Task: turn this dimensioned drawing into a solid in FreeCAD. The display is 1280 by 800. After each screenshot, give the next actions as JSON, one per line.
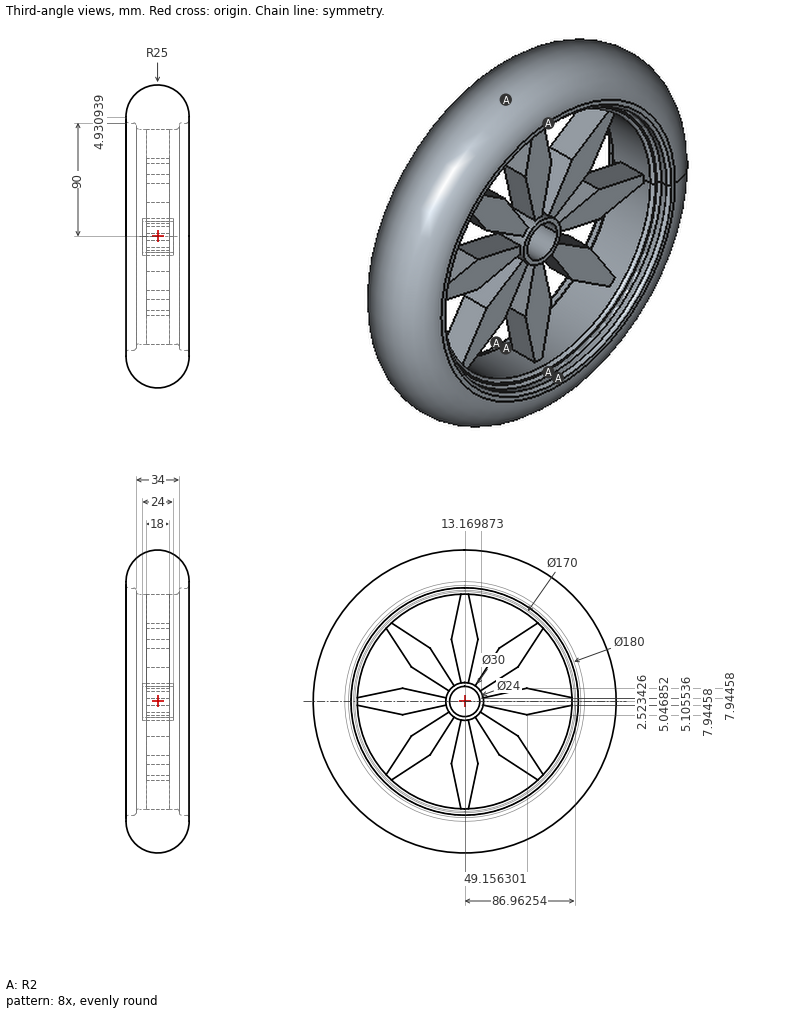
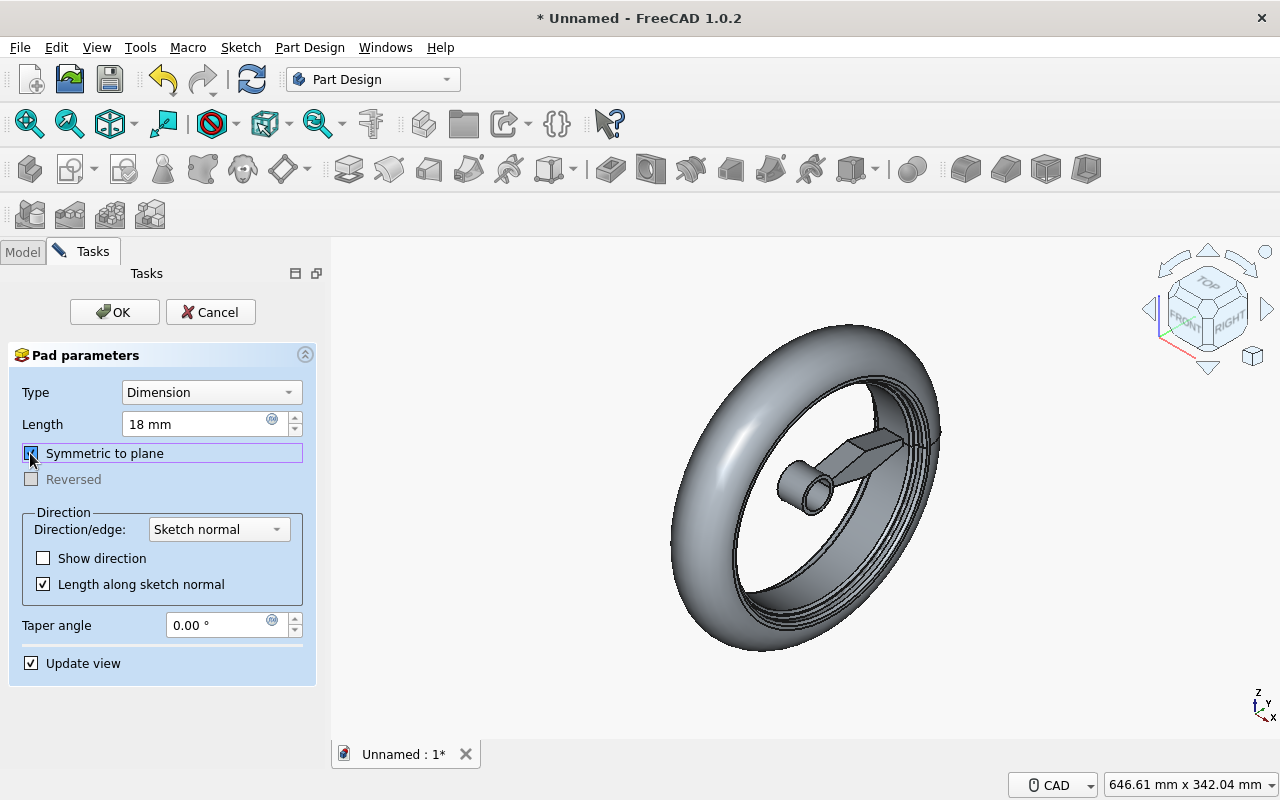
{"action": "left_click", "coordinate": [115, 312]}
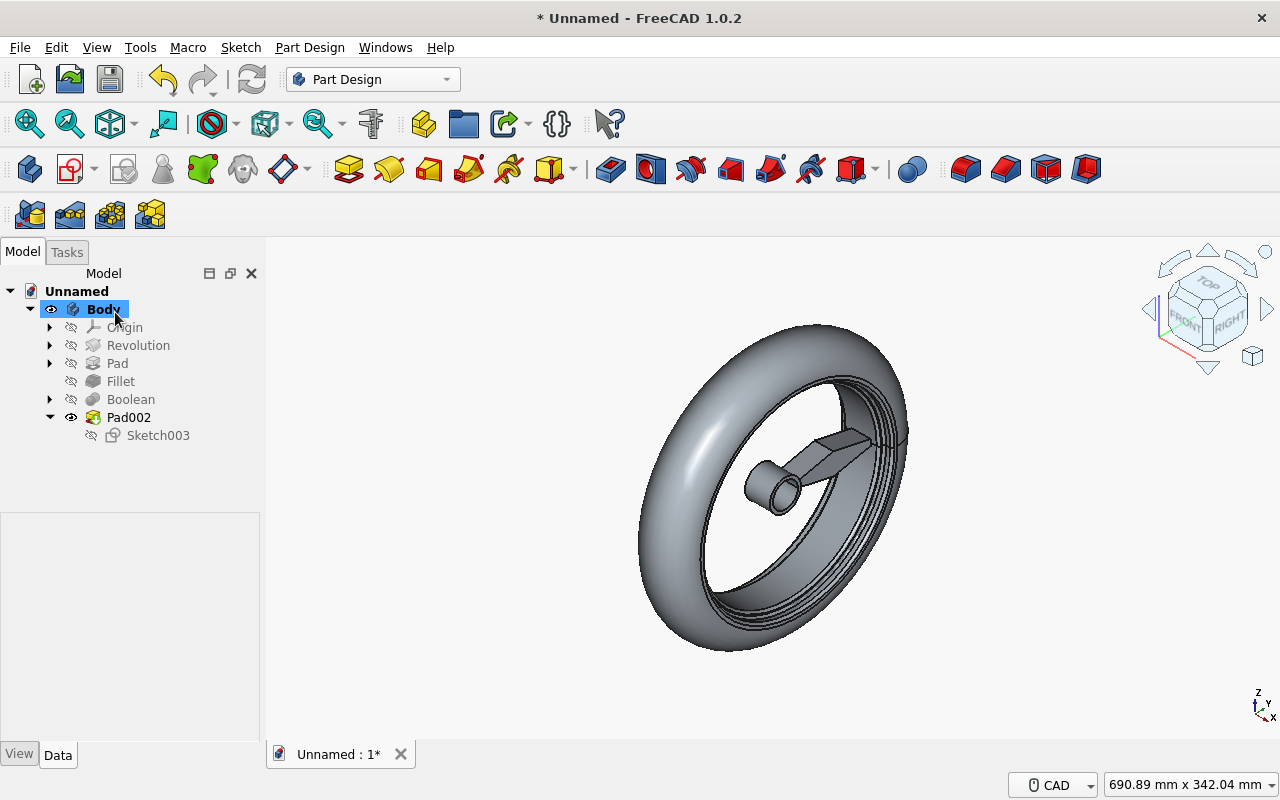
{"action": "left_click", "coordinate": [116, 417]}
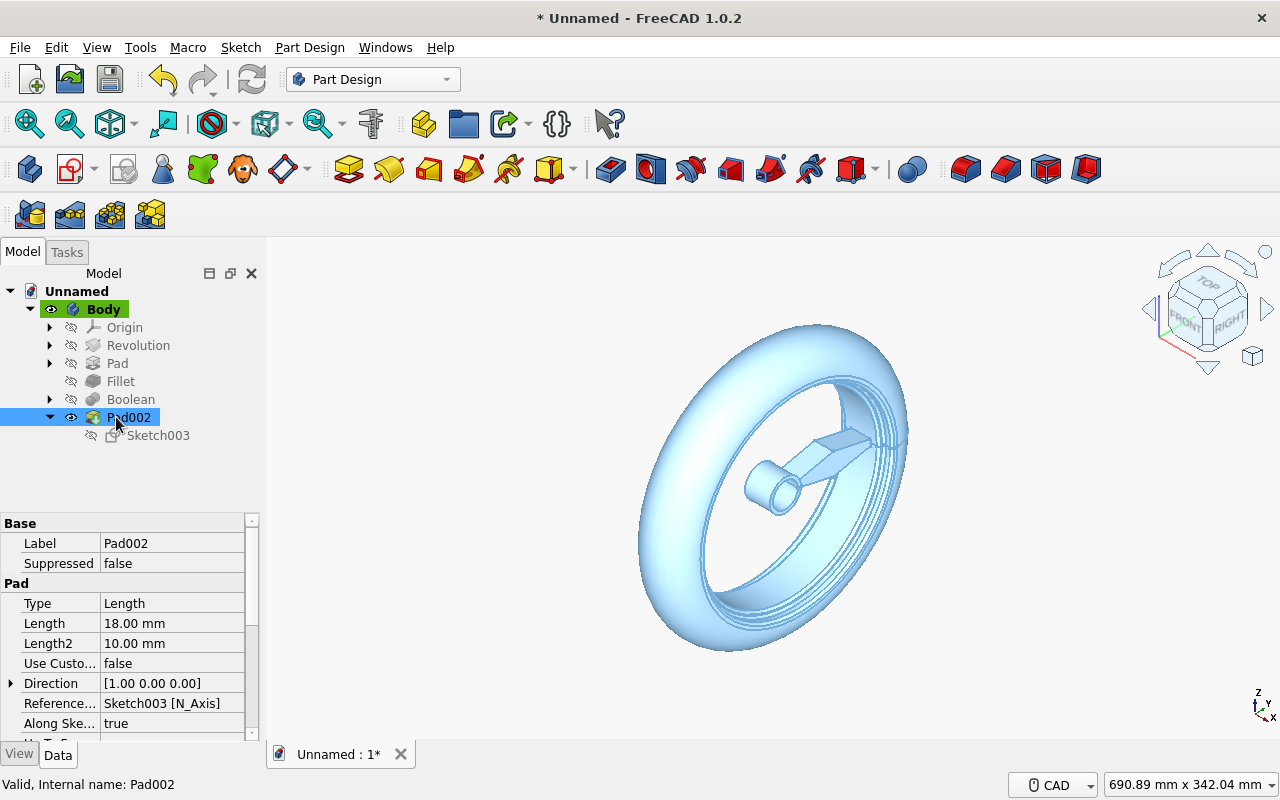
{"action": "left_click", "coordinate": [110, 214]}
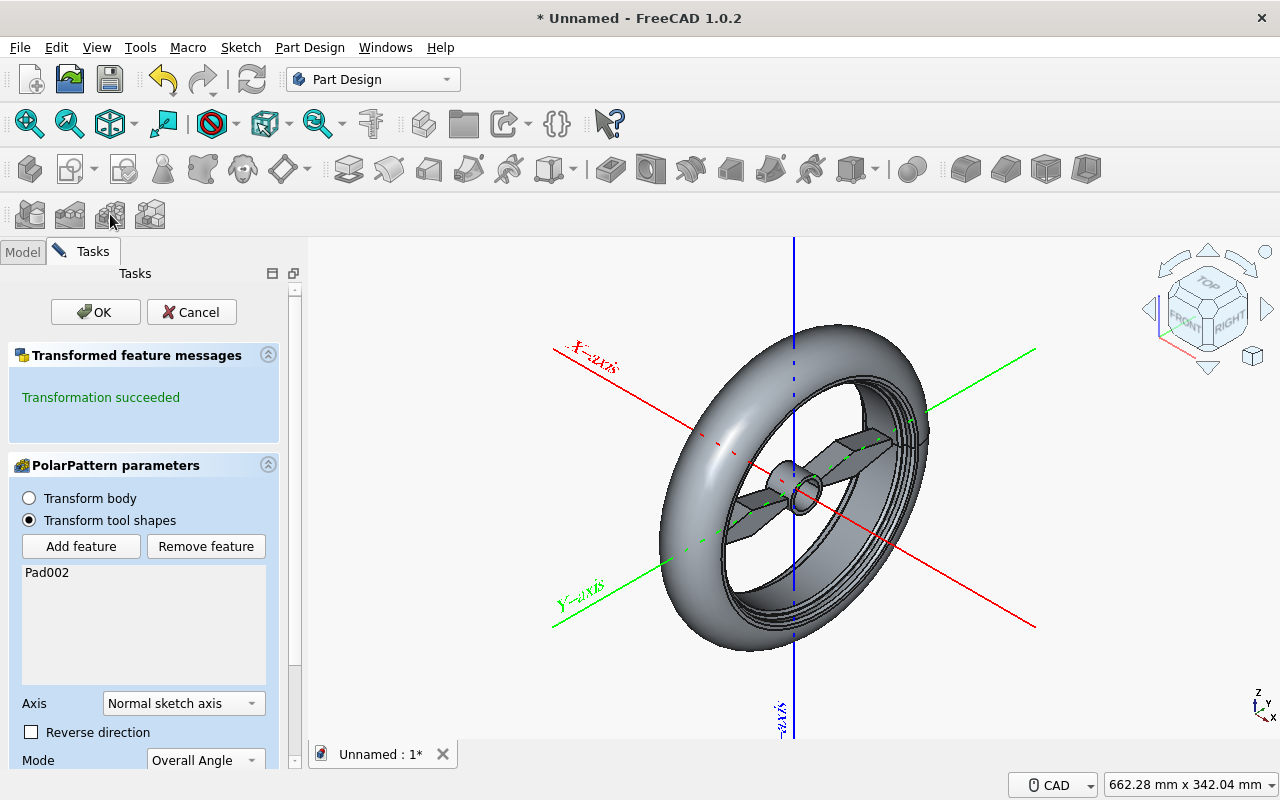
{"action": "left_click", "coordinate": [184, 704]}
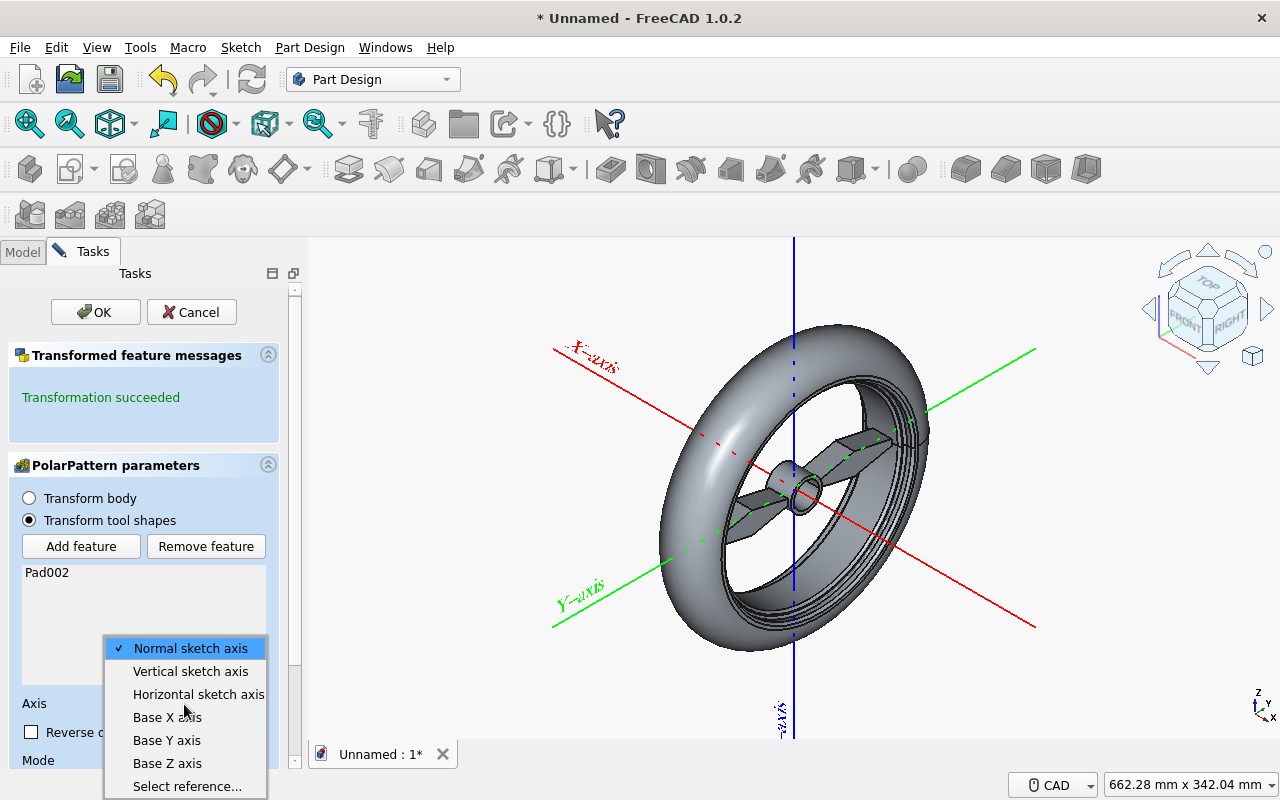
{"action": "left_click", "coordinate": [184, 718]}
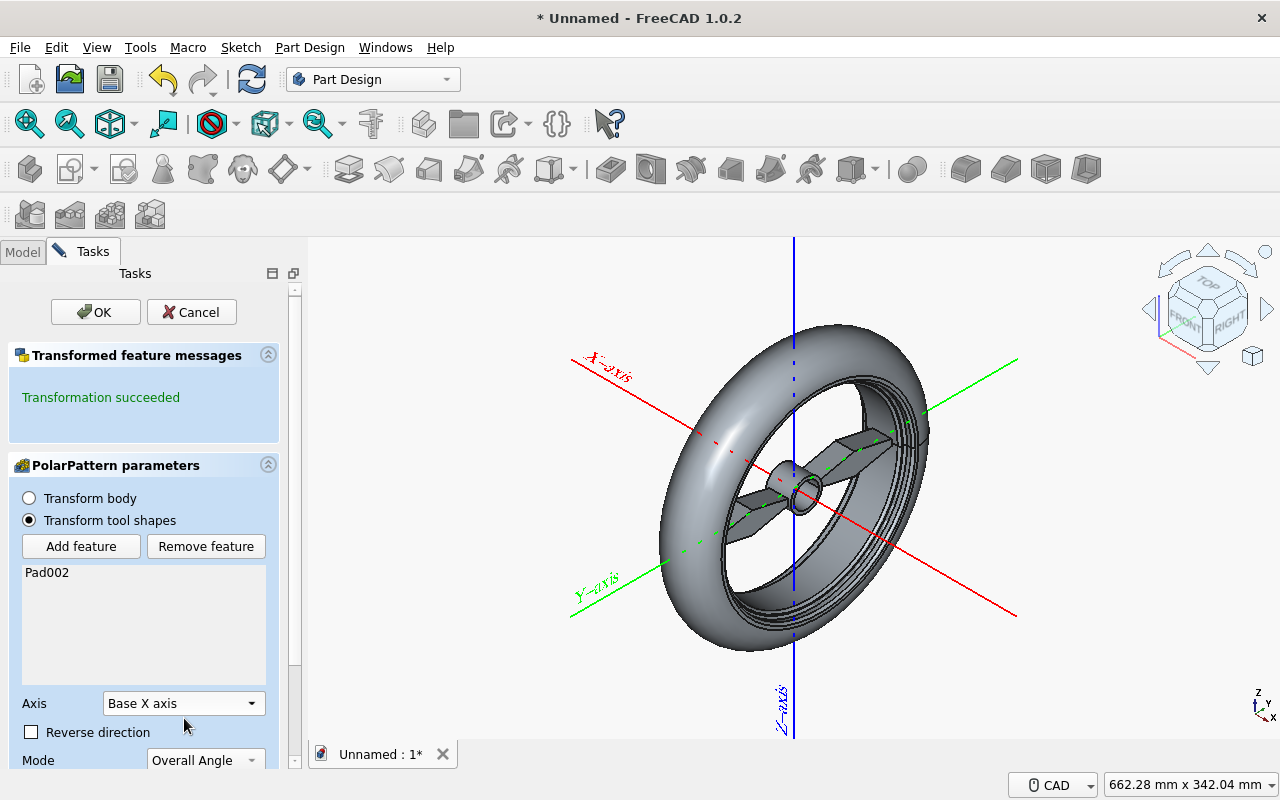
{"action": "scroll", "coordinate": [295, 526], "scroll_direction": "down", "scroll_amount": 3}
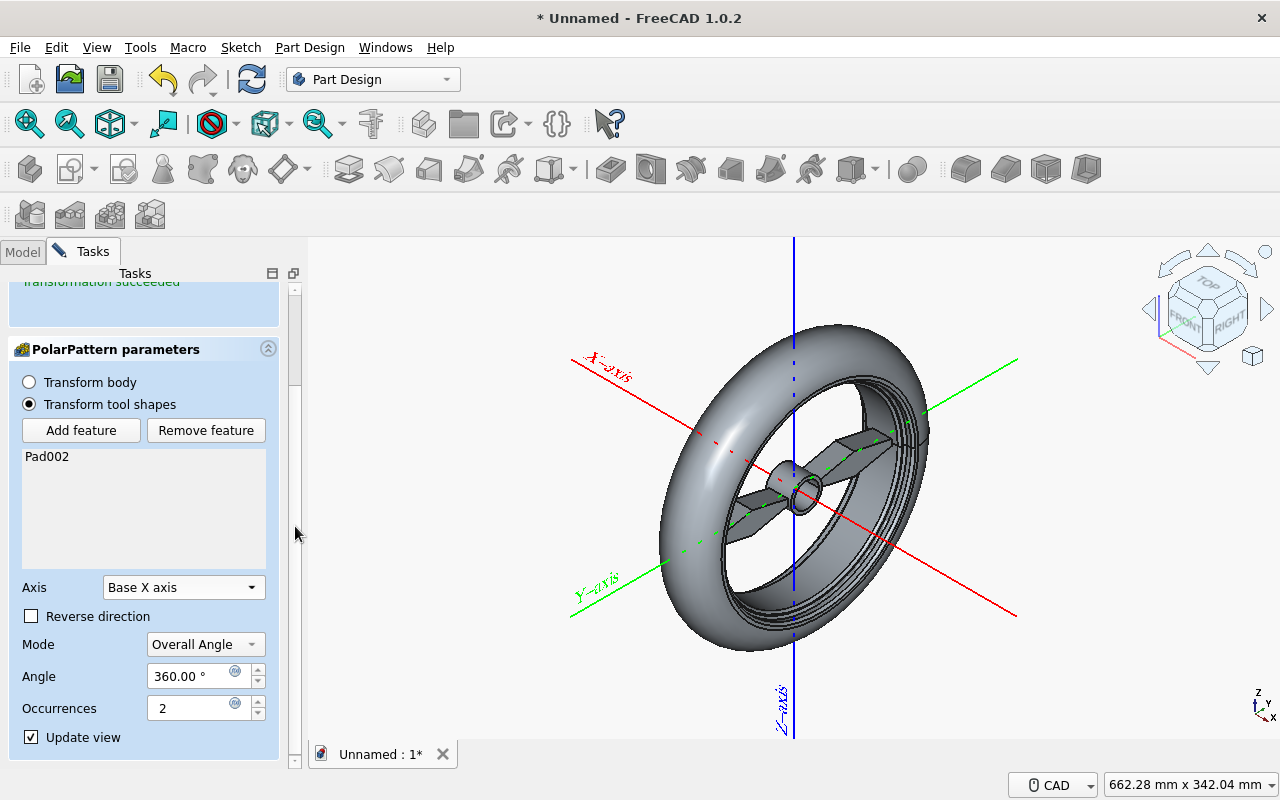
{"action": "triple_click", "coordinate": [198, 708]}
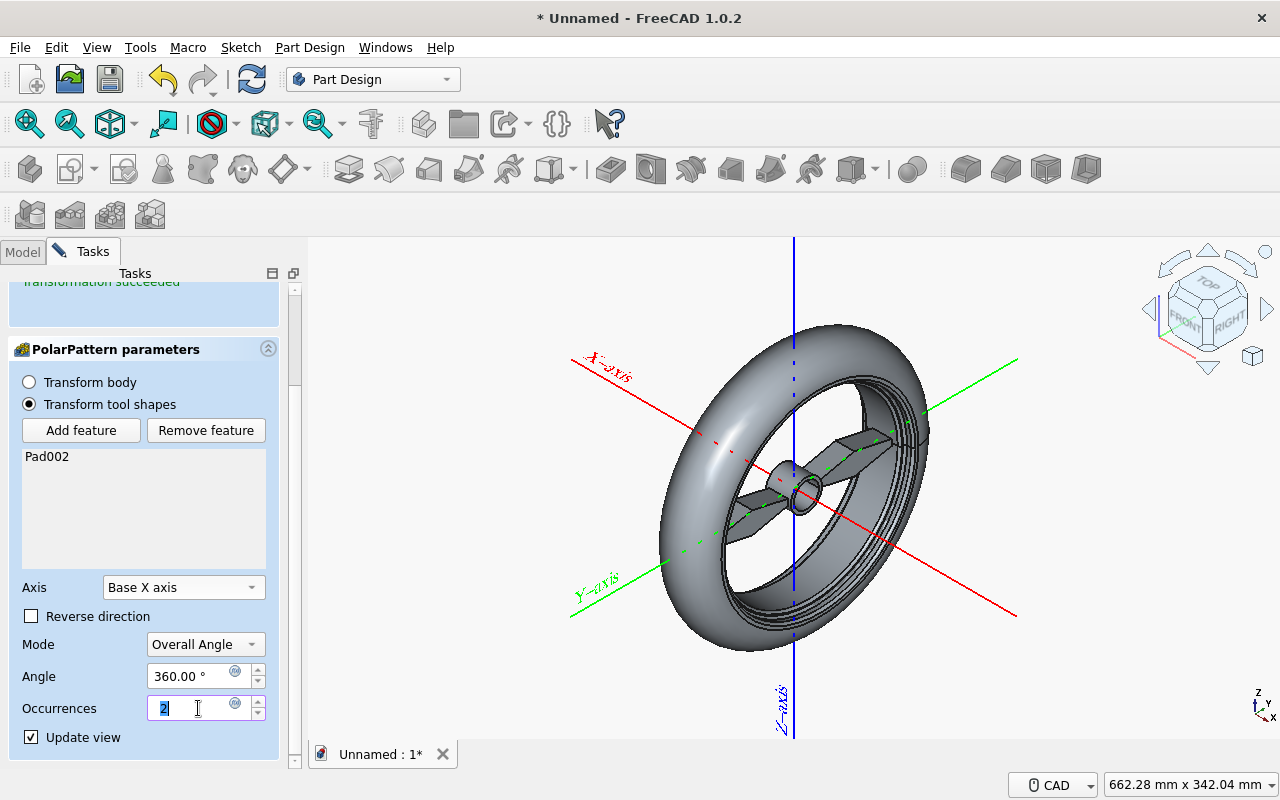
{"action": "type", "text": "8"}
{"action": "key", "text": "Tab"}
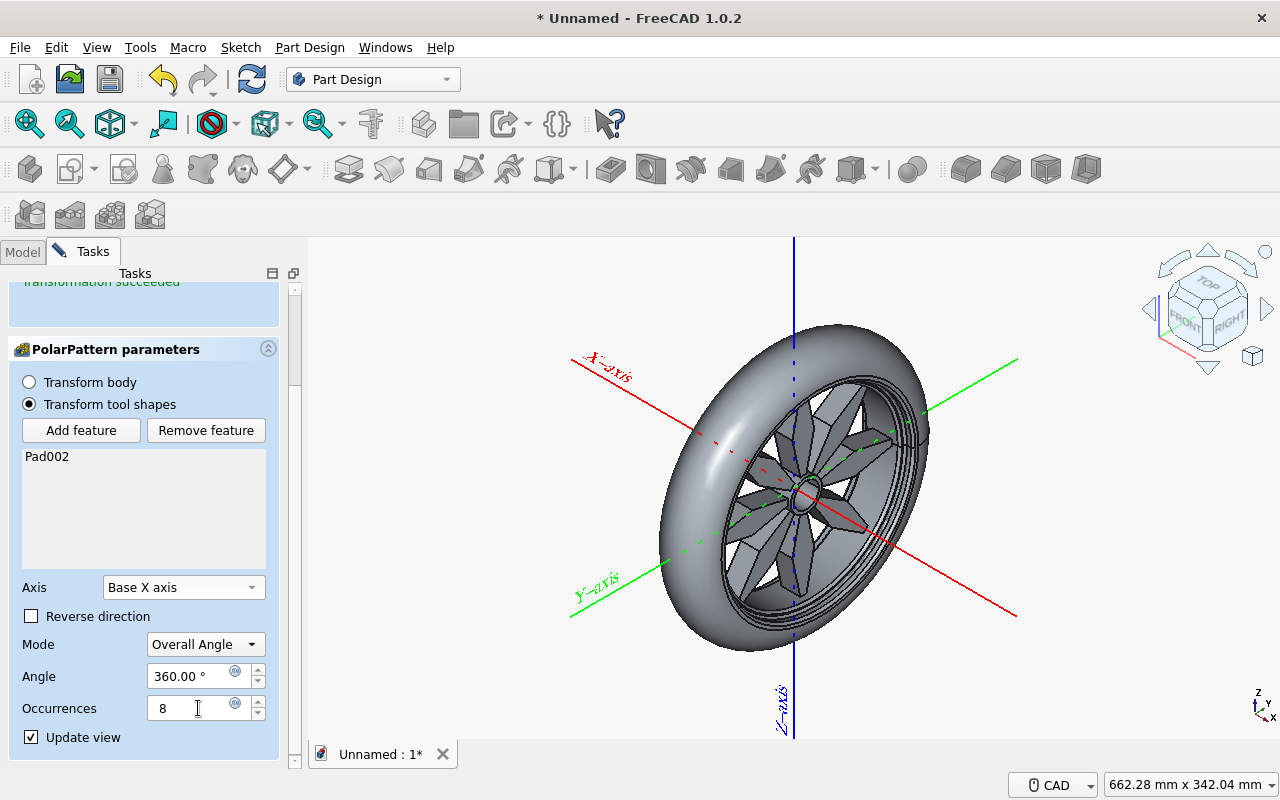
{"action": "scroll", "coordinate": [295, 526], "scroll_direction": "up", "scroll_amount": 3}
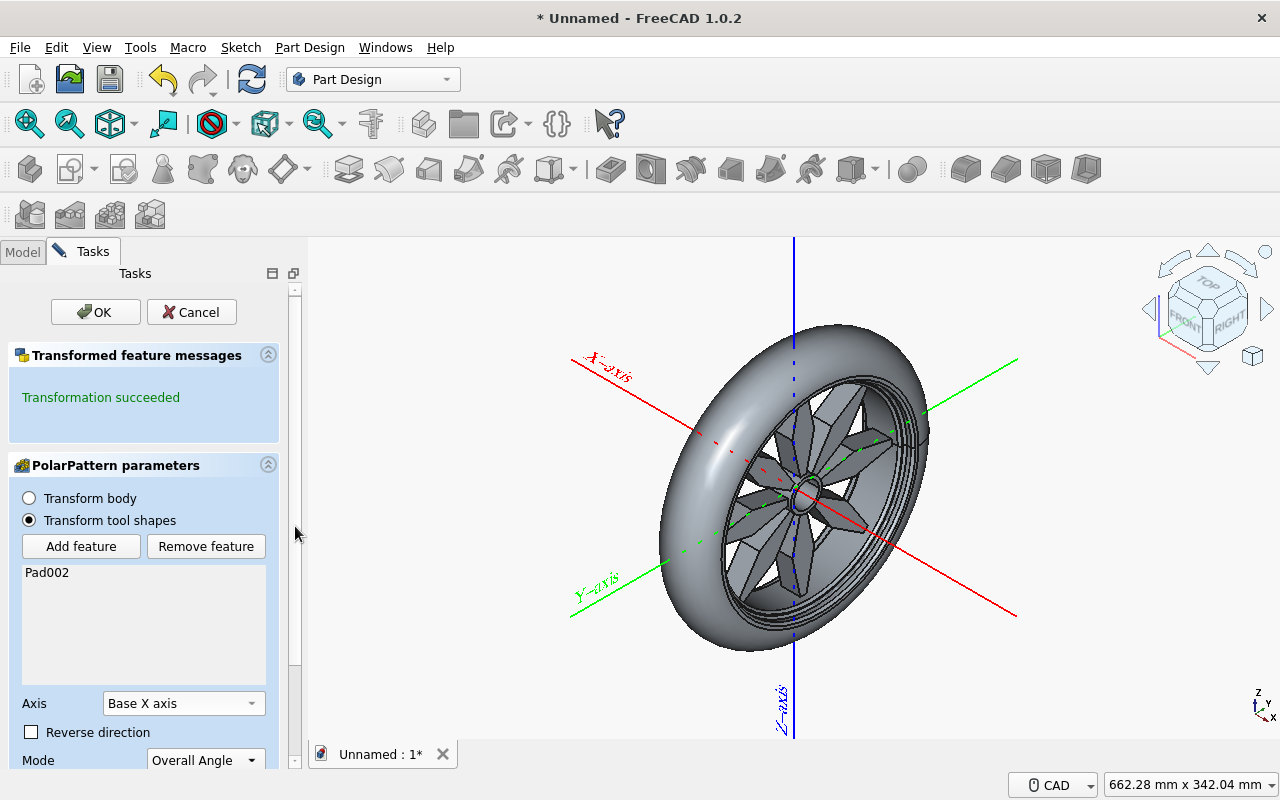
{"action": "left_click", "coordinate": [96, 312]}